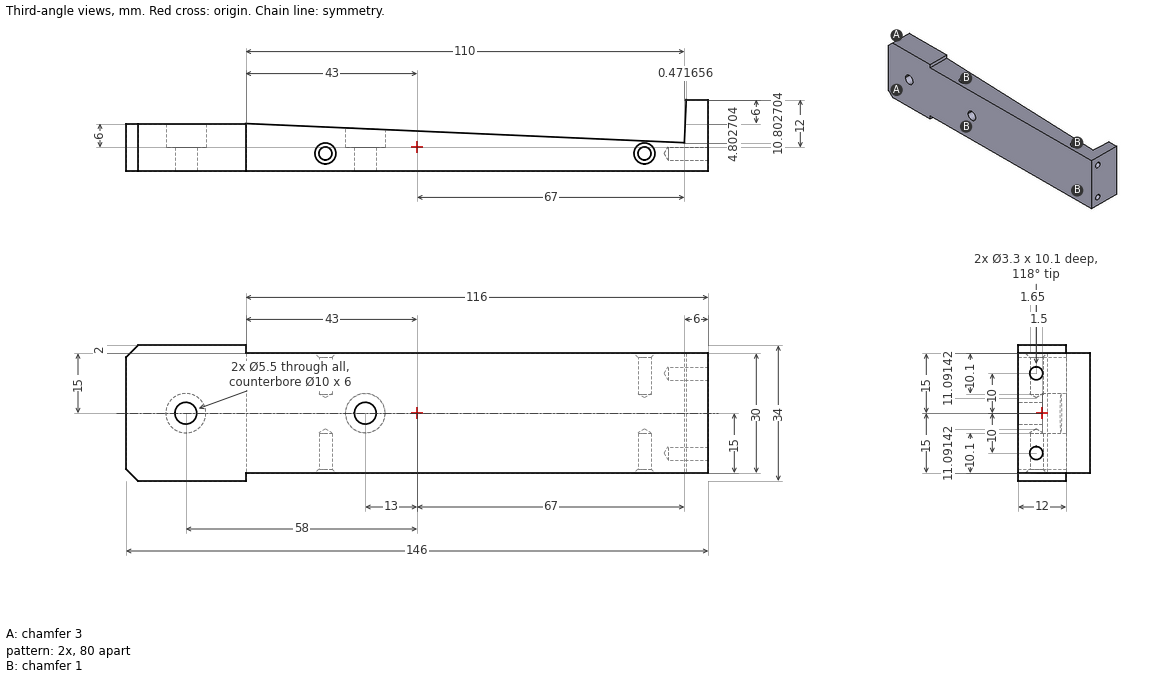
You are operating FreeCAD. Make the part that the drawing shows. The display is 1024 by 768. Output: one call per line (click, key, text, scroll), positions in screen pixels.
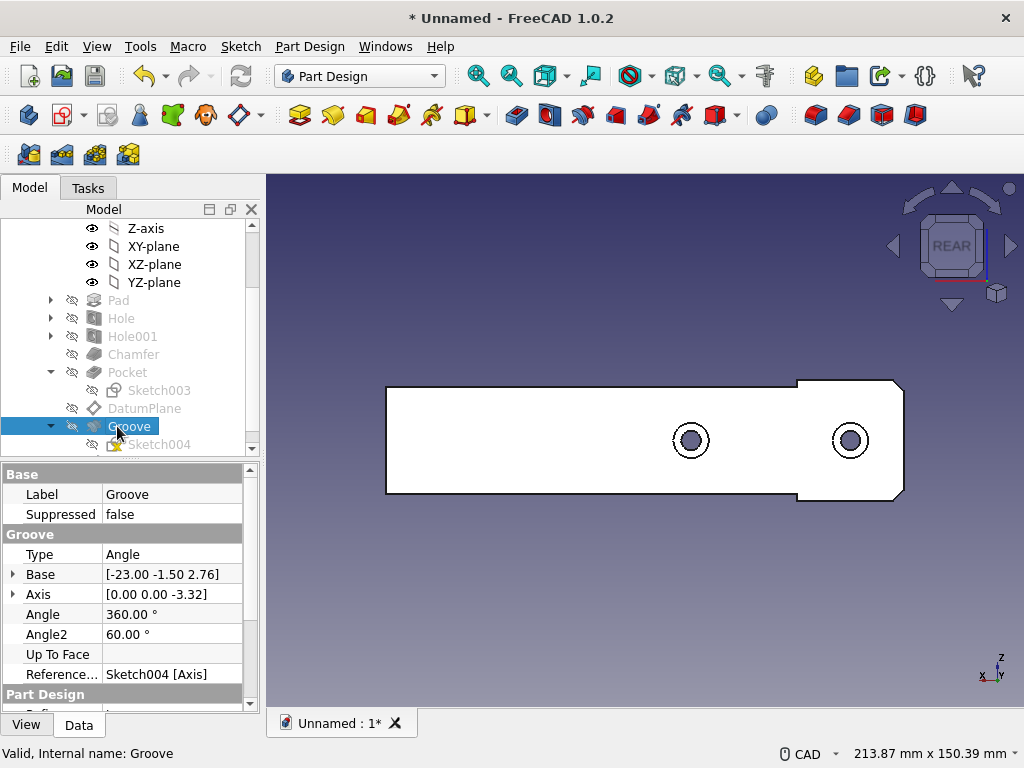
click(29, 154)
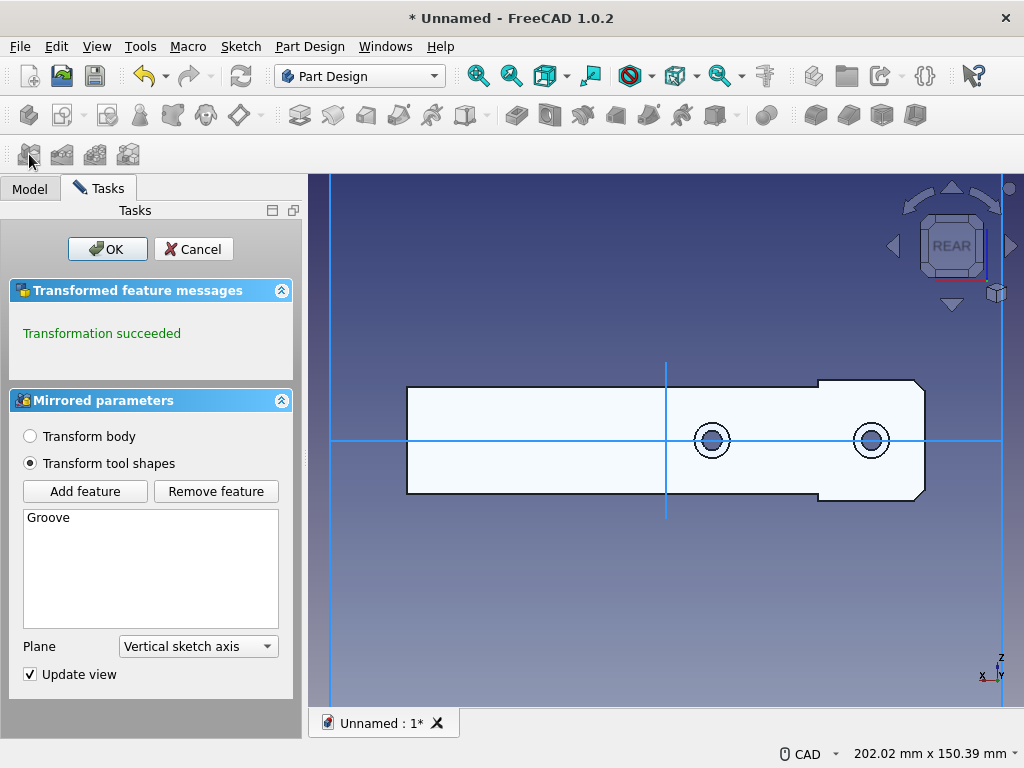
click(199, 646)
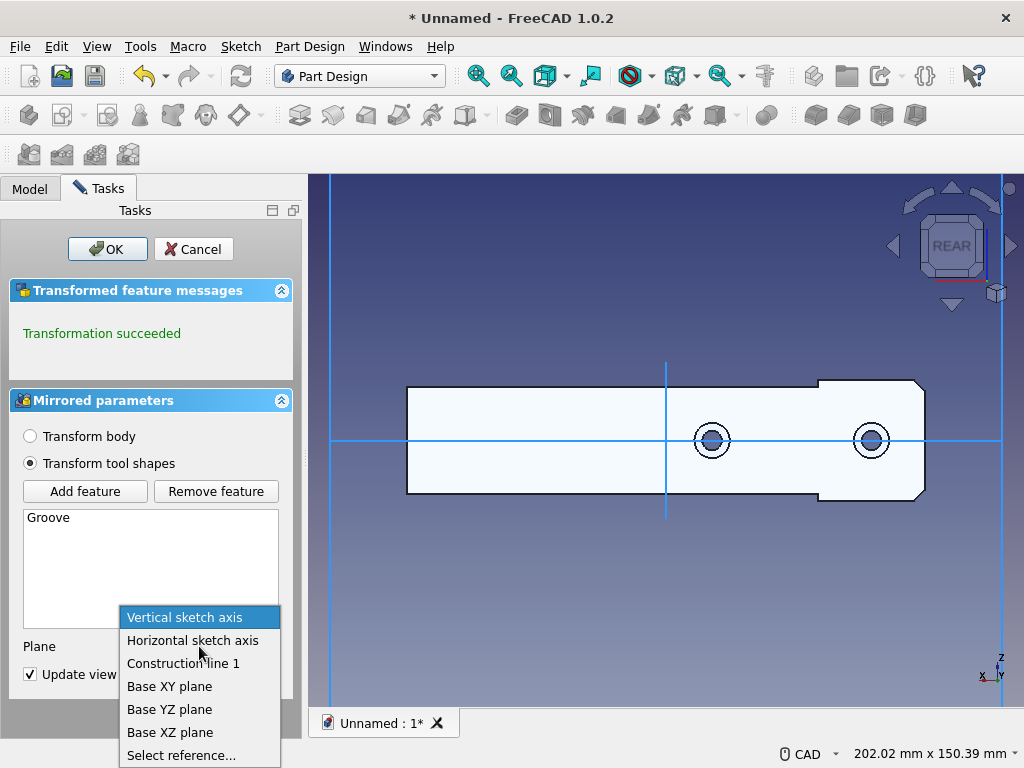
click(198, 686)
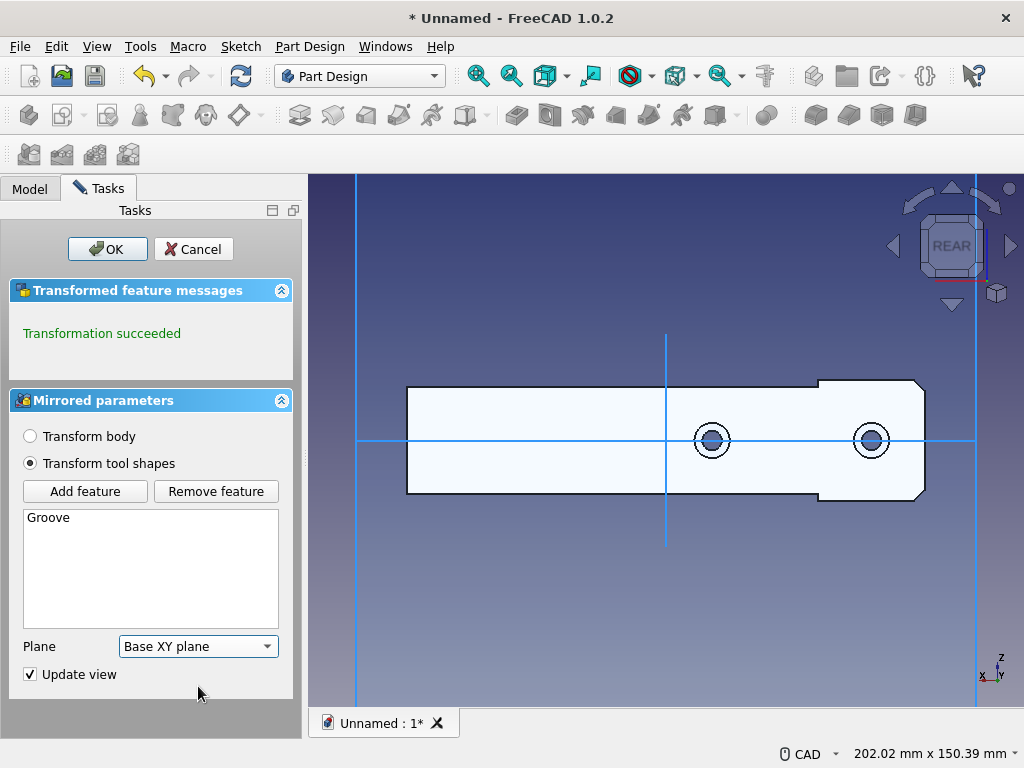
click(108, 249)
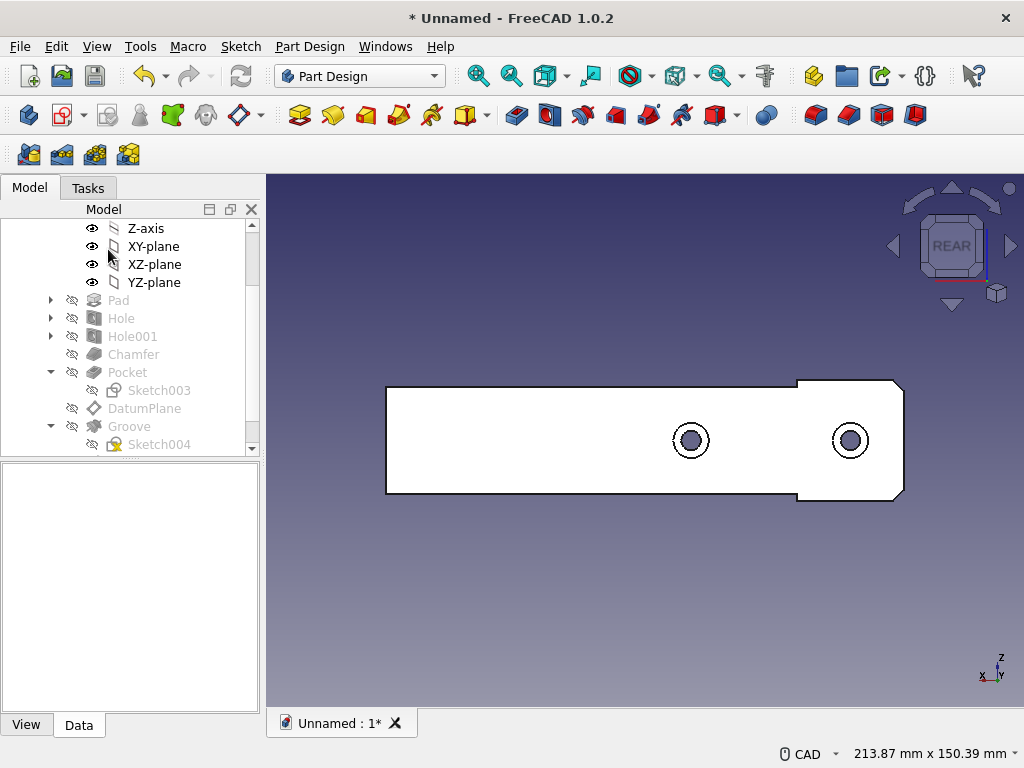
scroll(161, 332, down, 3)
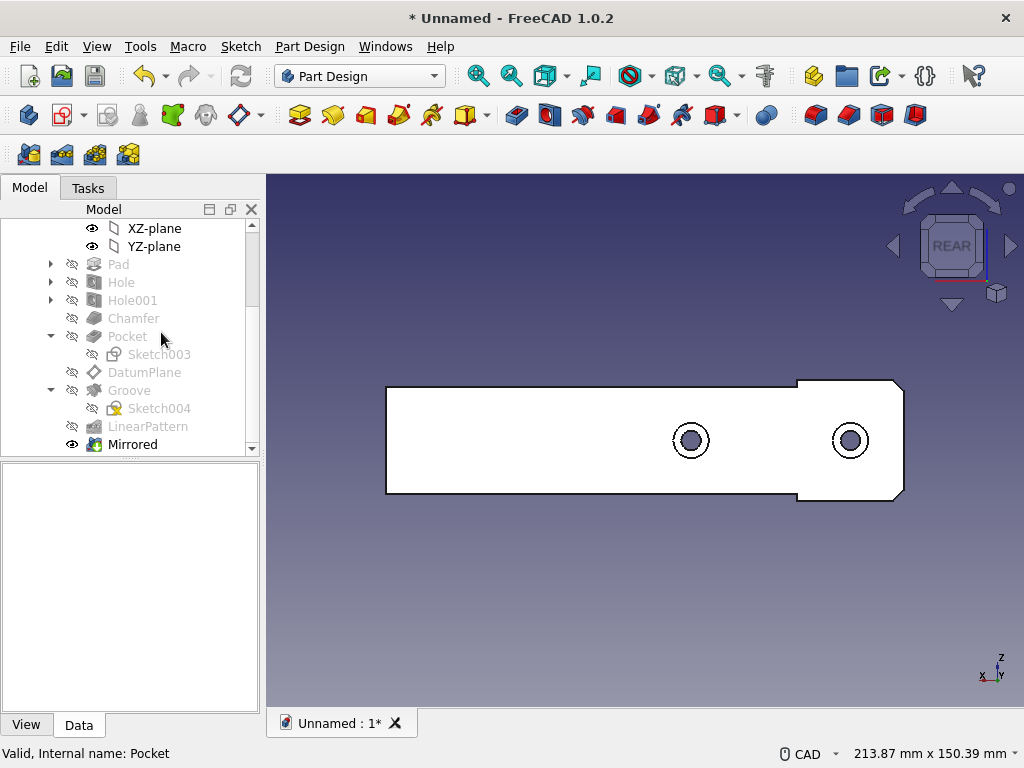
scroll(161, 332, up, 15)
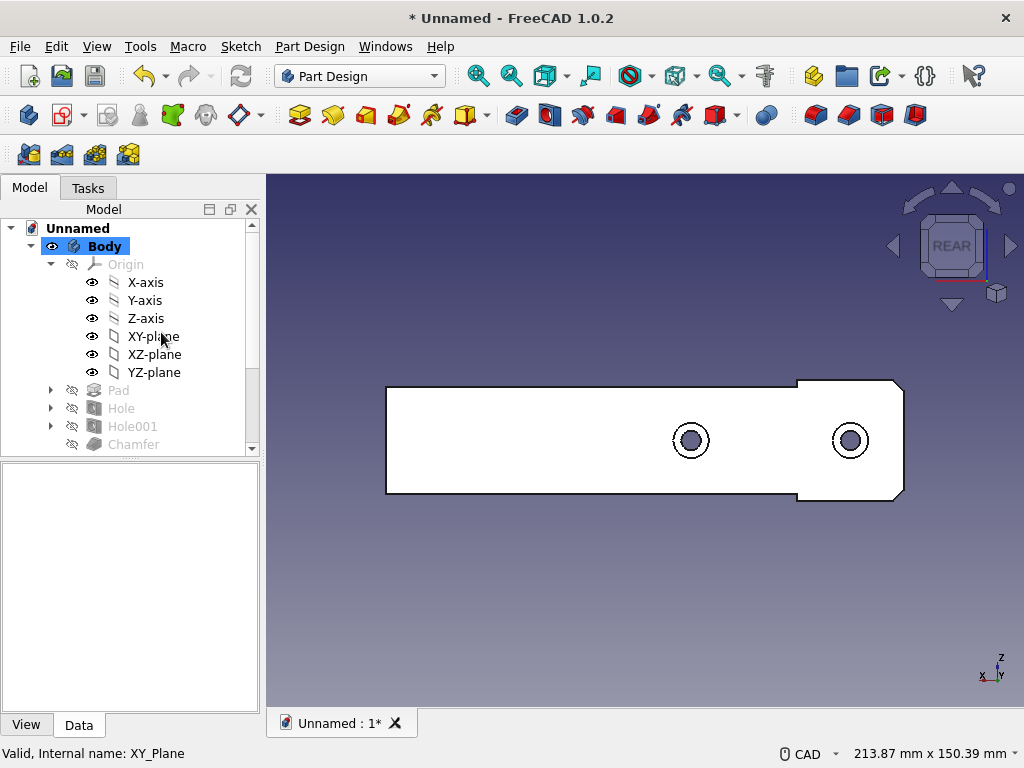
click(137, 372)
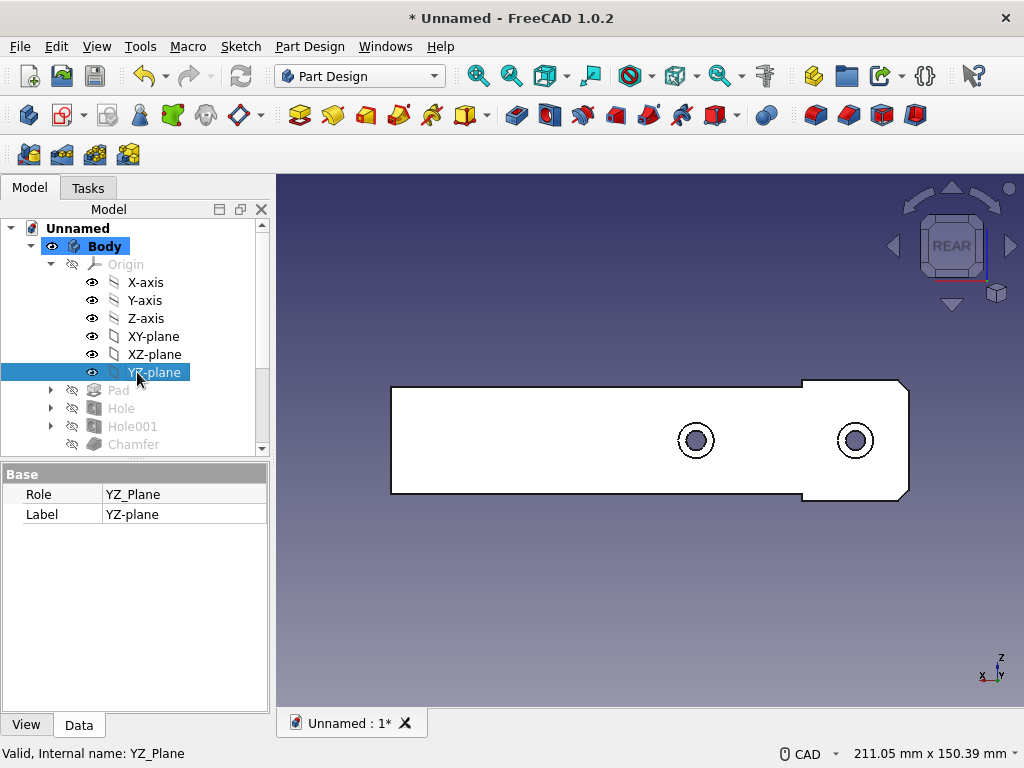
click(238, 116)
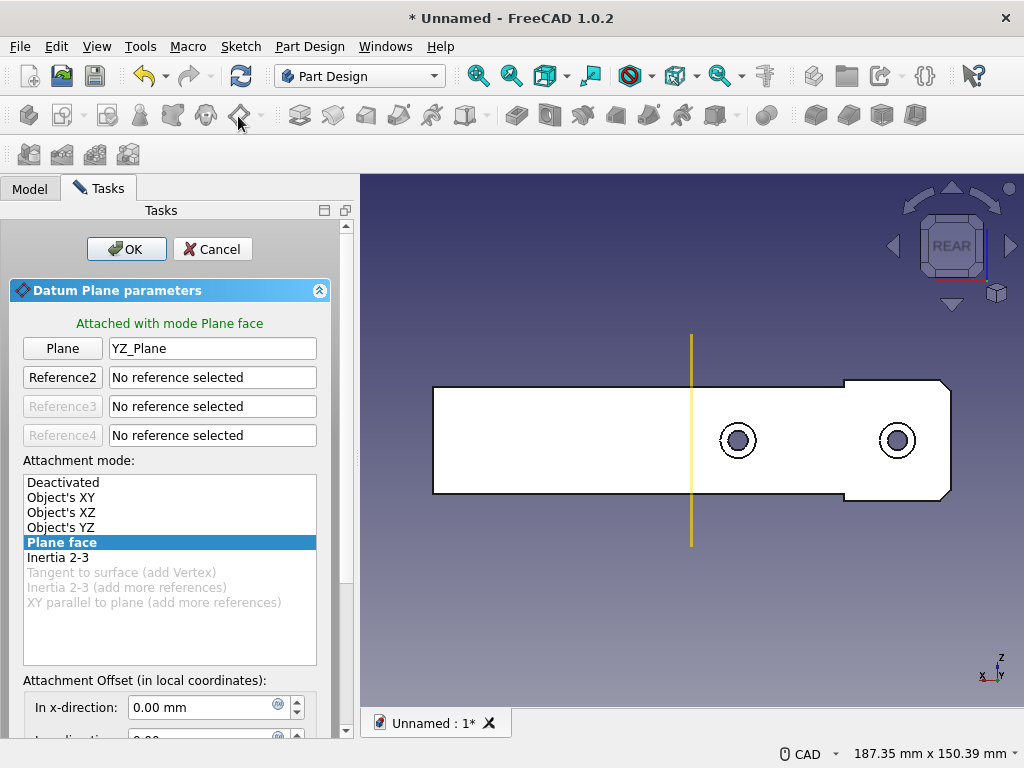
scroll(346, 479, down, 2)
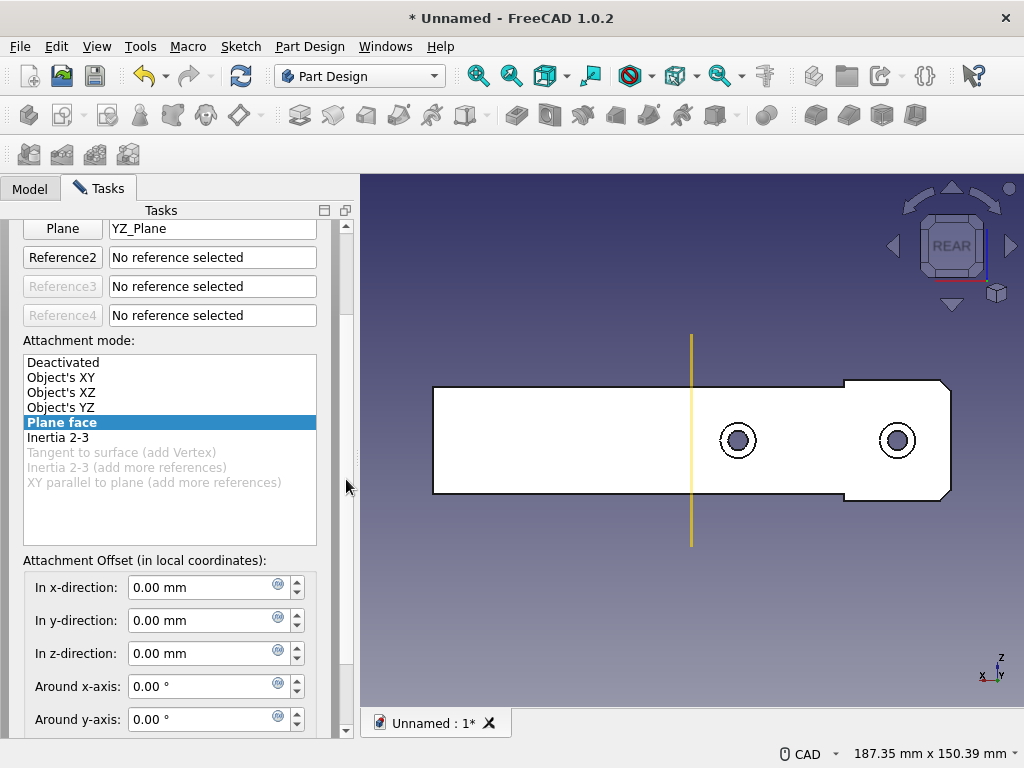
triple_click(210, 654)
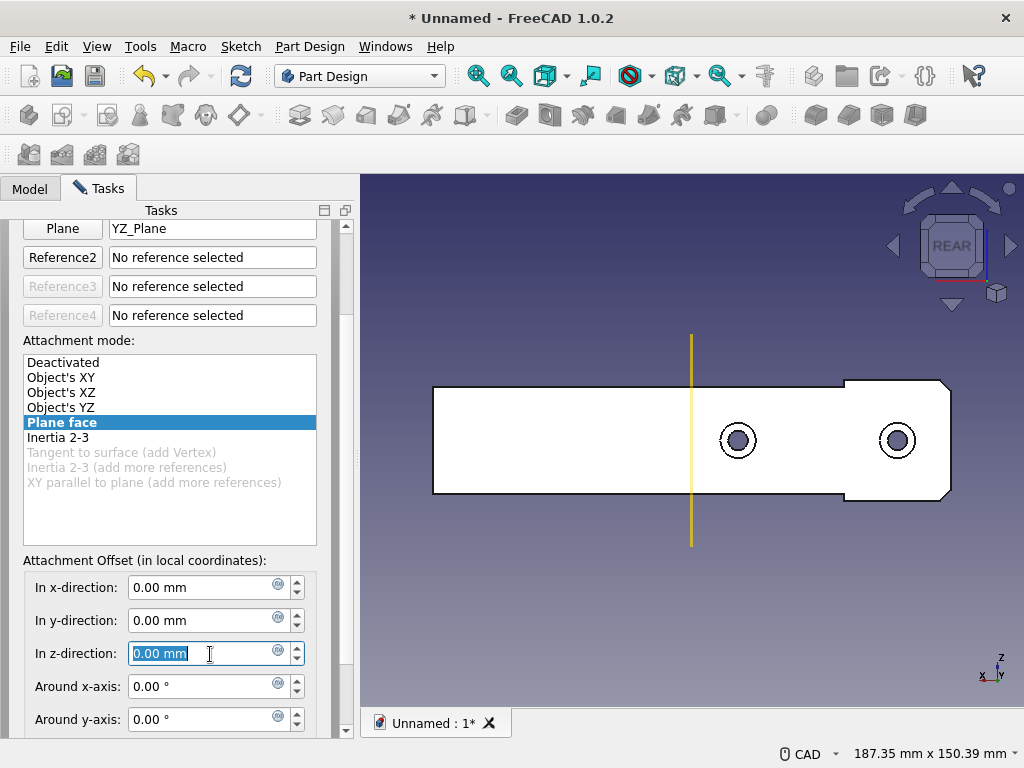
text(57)
key(Tab)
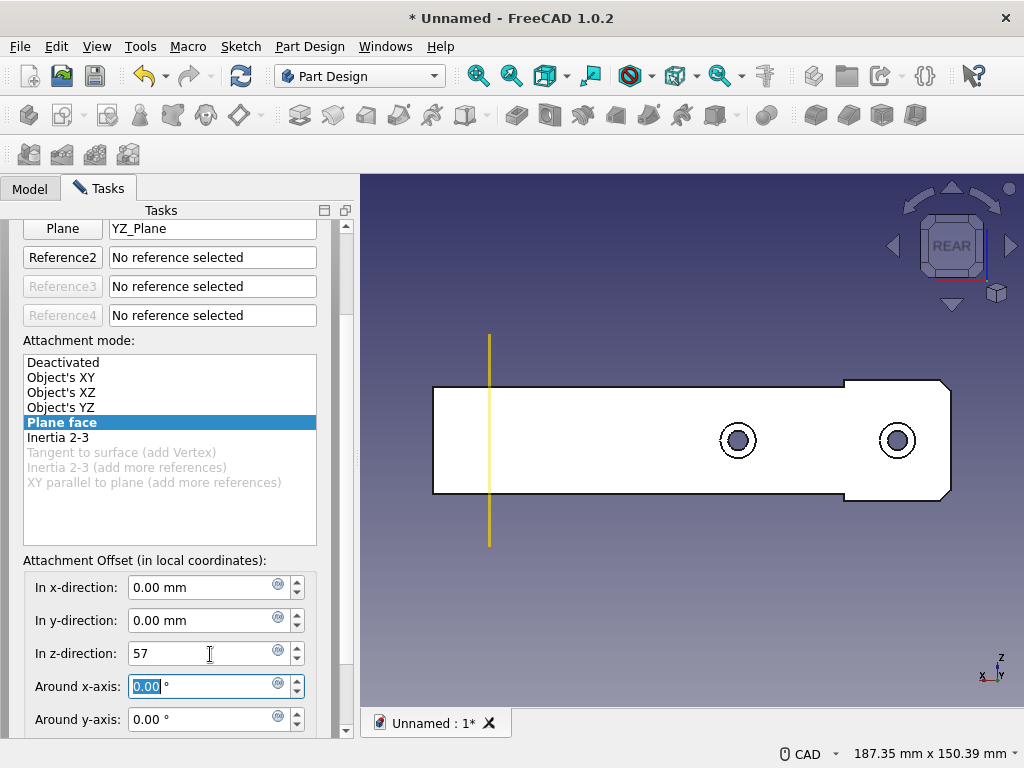
scroll(346, 479, up, 3)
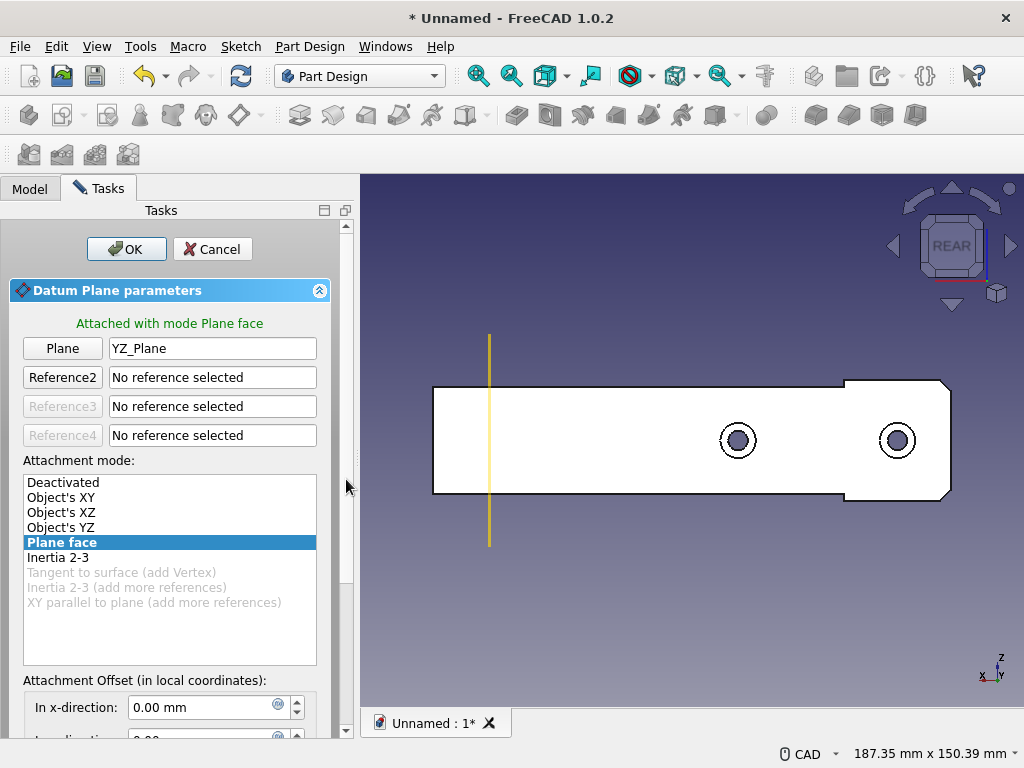
click(127, 249)